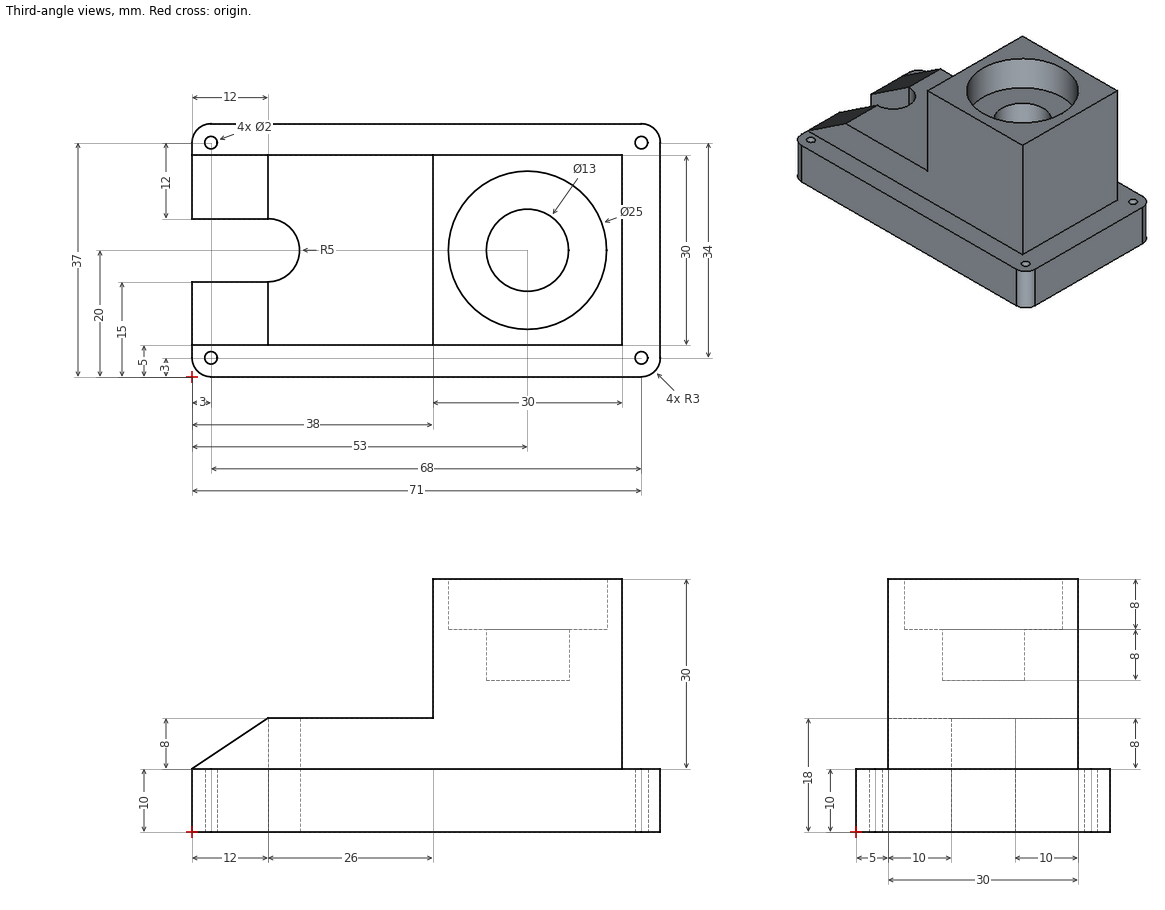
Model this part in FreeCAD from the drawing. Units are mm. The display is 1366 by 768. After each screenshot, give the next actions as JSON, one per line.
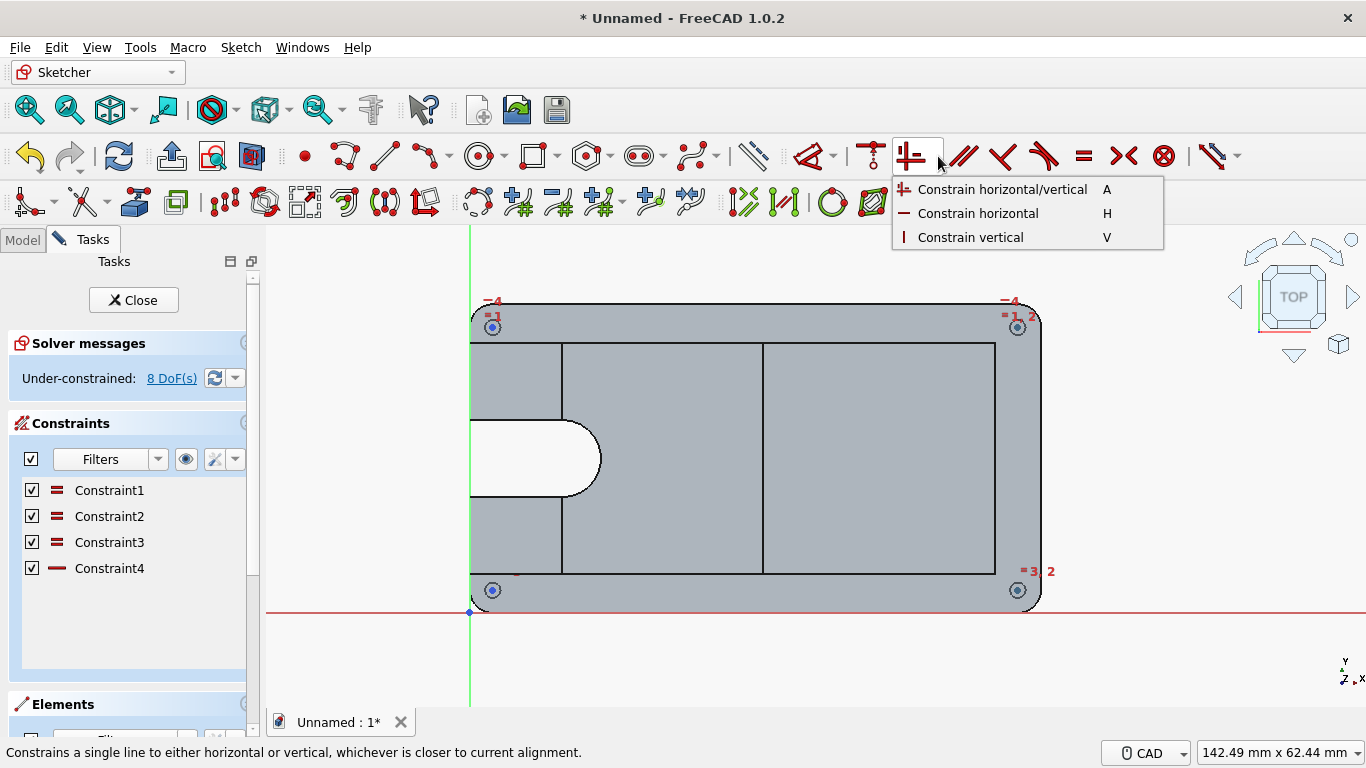
{"action": "left_click", "coordinate": [1028, 237]}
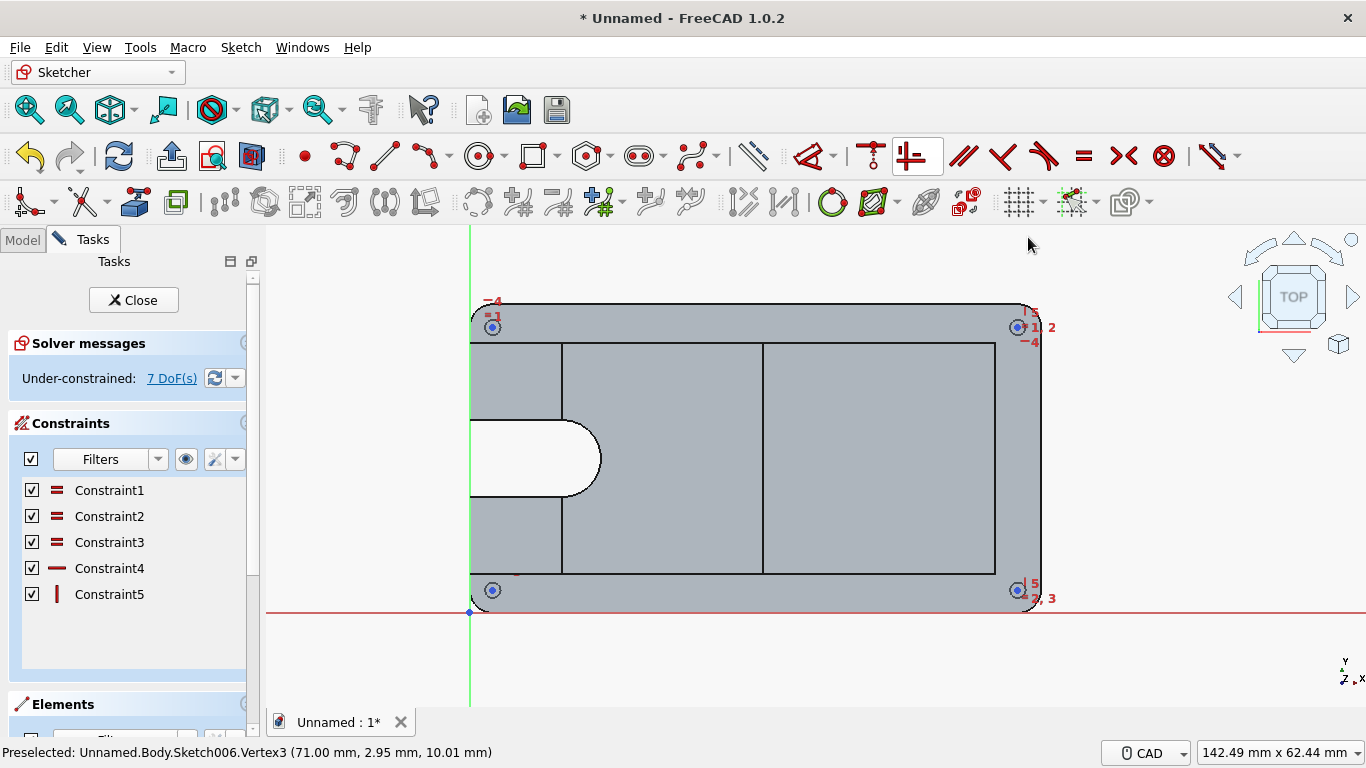
{"action": "left_click", "coordinate": [493, 328]}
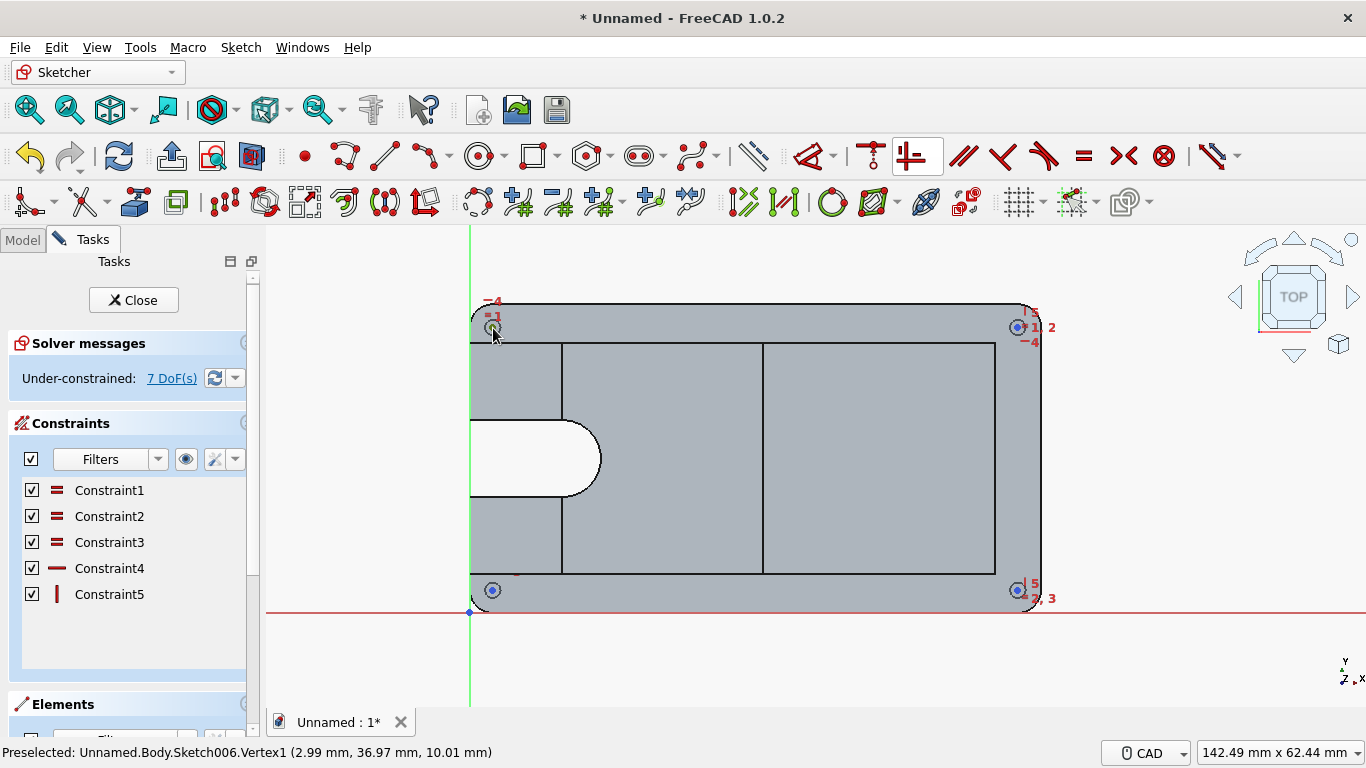
{"action": "left_click", "coordinate": [493, 590]}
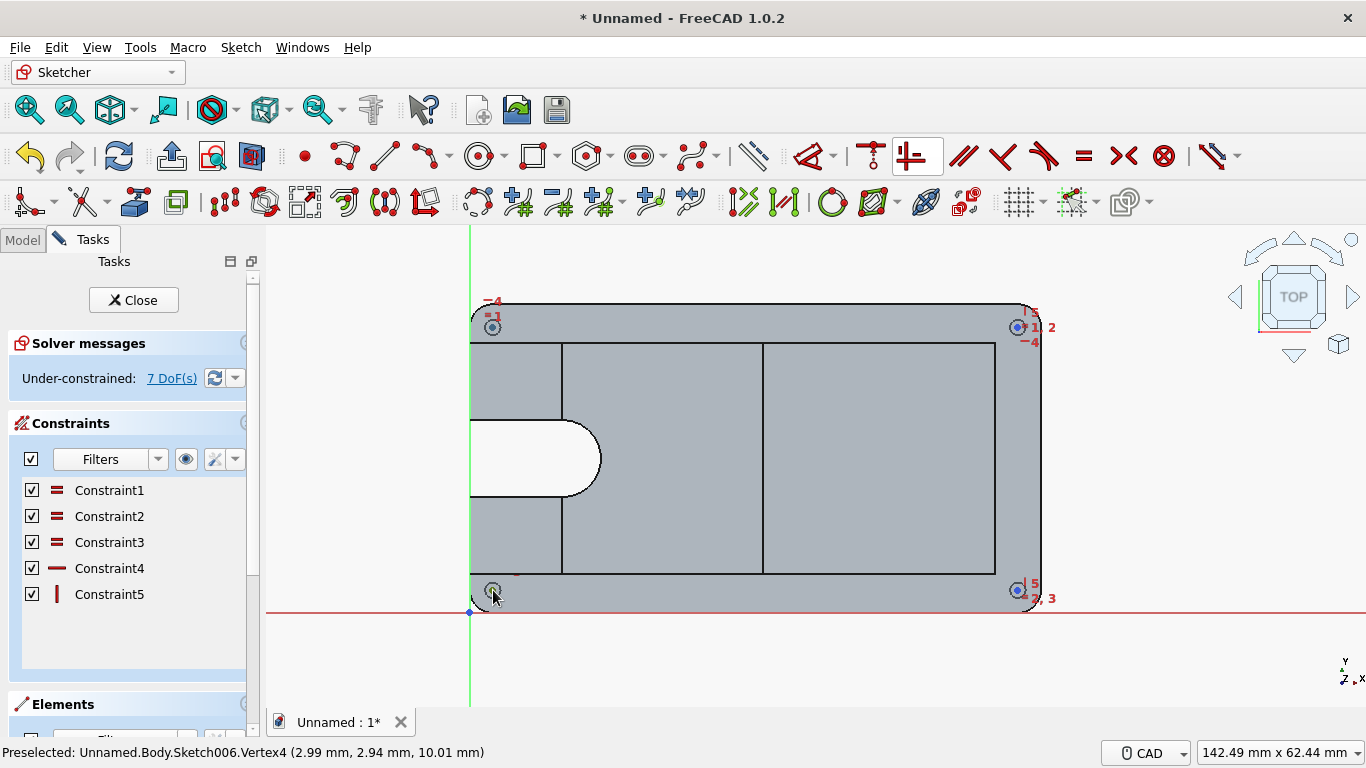
{"action": "left_click", "coordinate": [938, 156]}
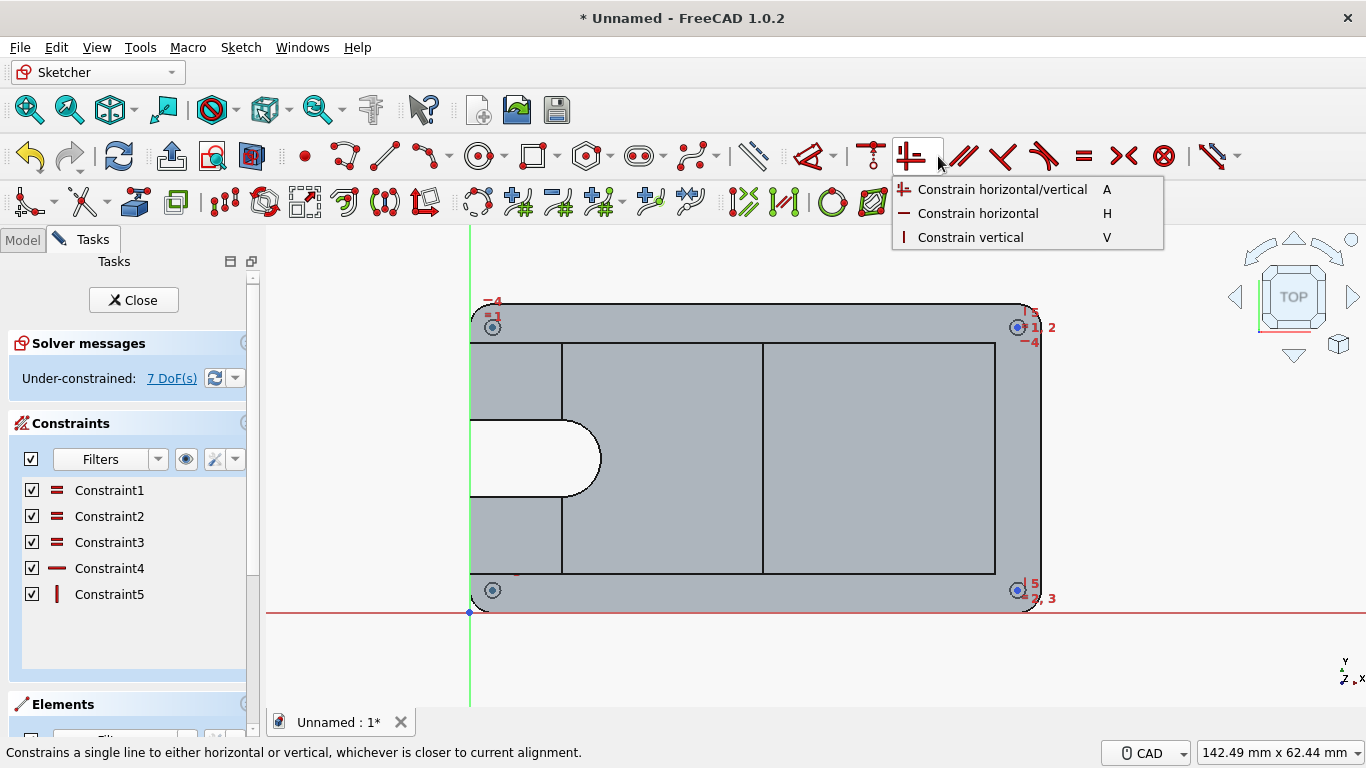
{"action": "left_click", "coordinate": [1028, 237]}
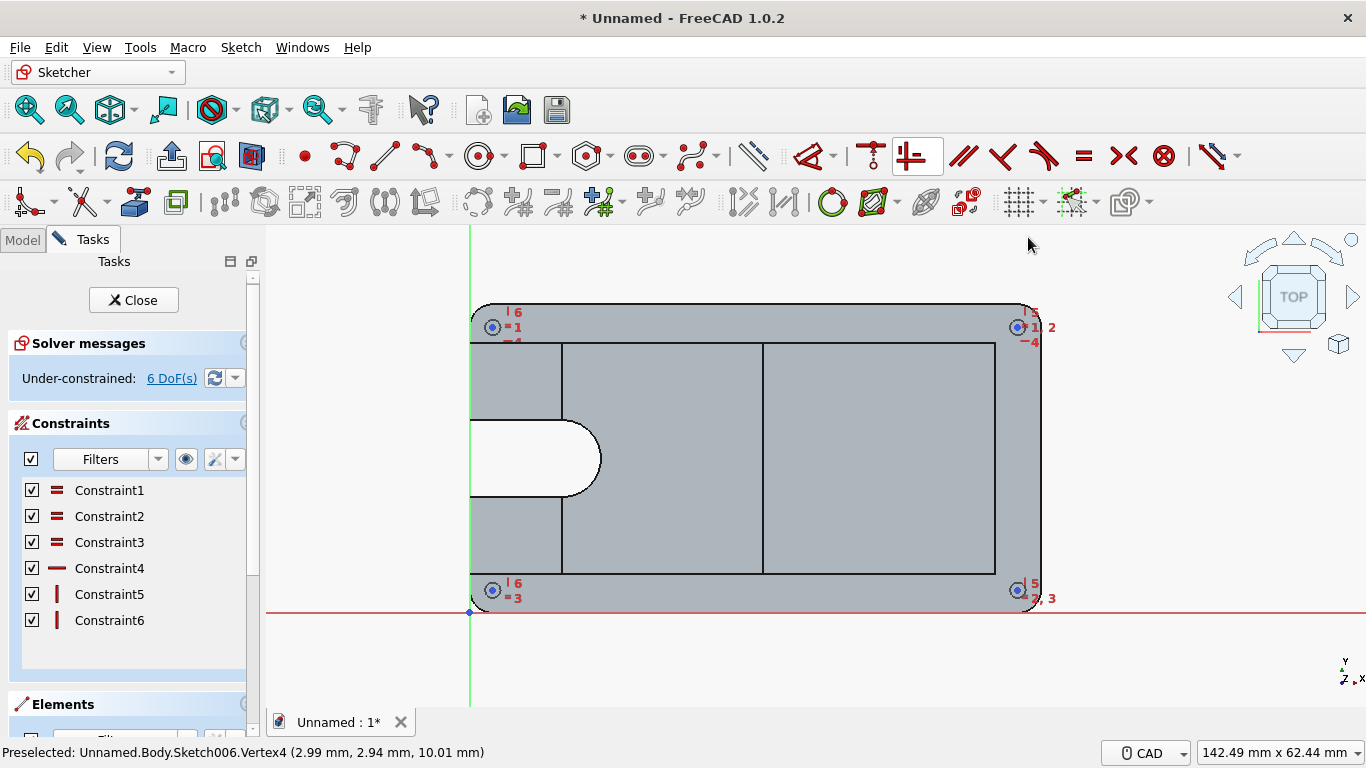
{"action": "left_click", "coordinate": [1018, 590]}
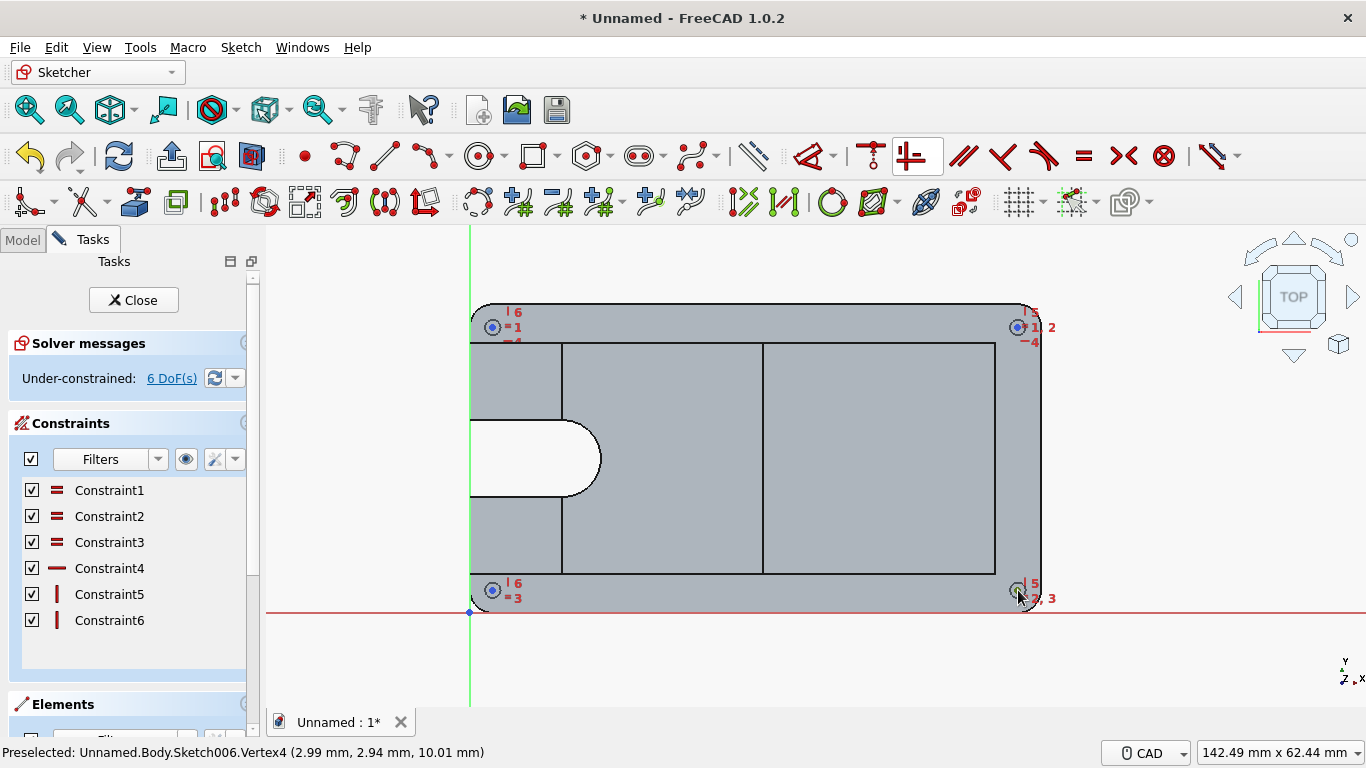
{"action": "left_click", "coordinate": [493, 590]}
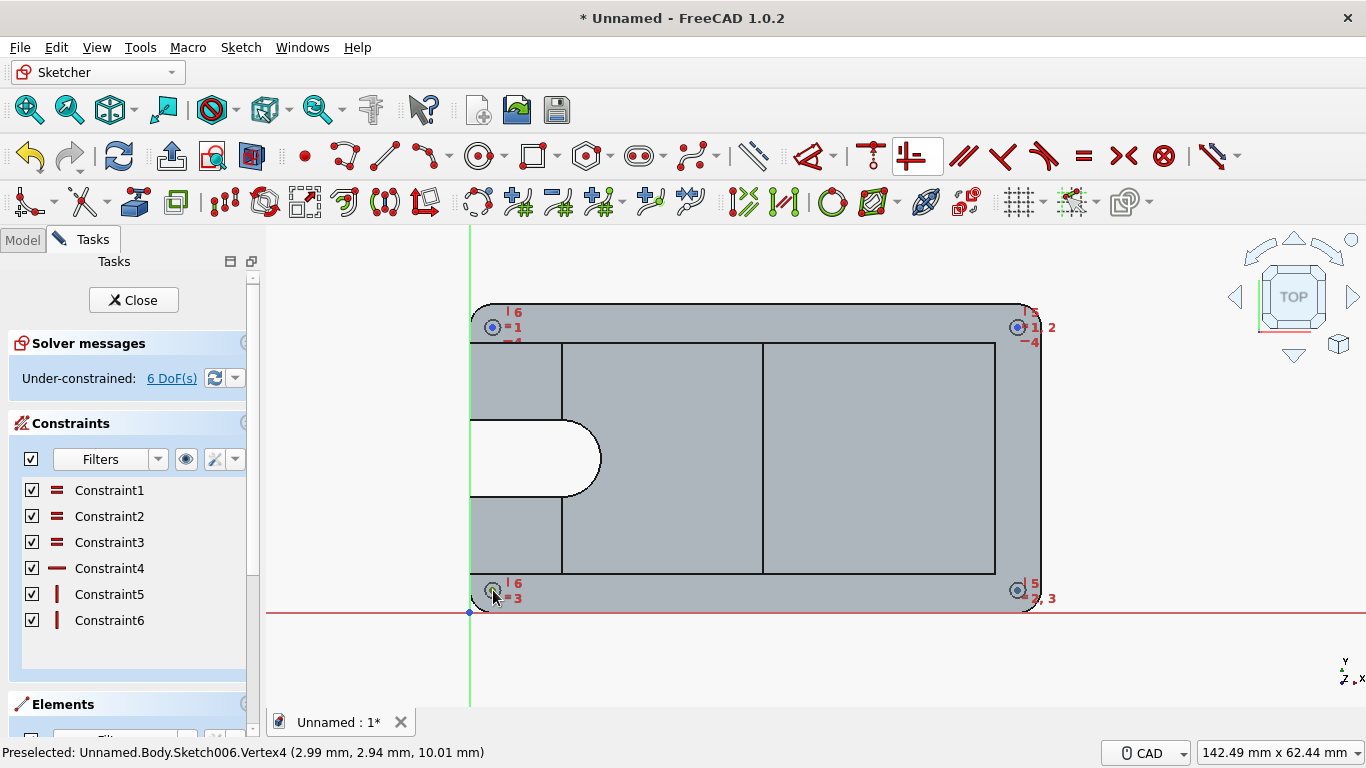
{"action": "key", "text": "h"}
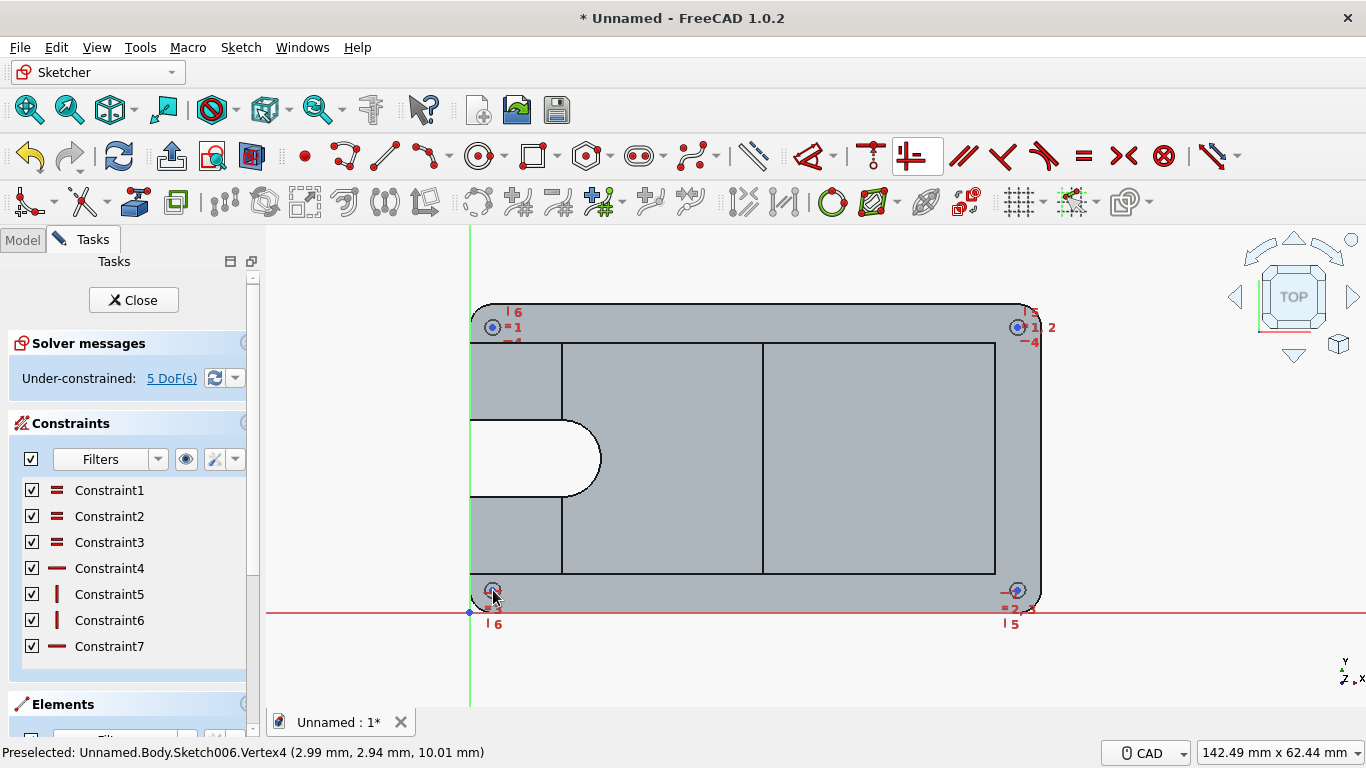
{"action": "key", "text": "d"}